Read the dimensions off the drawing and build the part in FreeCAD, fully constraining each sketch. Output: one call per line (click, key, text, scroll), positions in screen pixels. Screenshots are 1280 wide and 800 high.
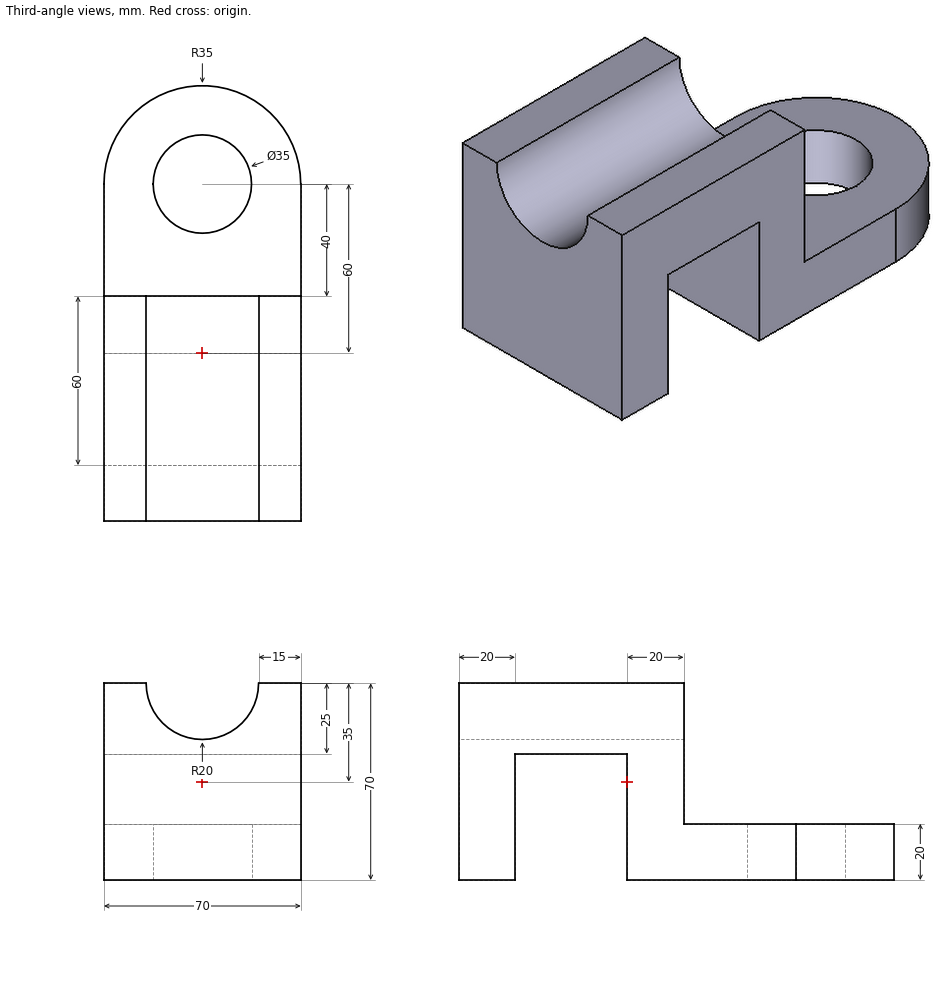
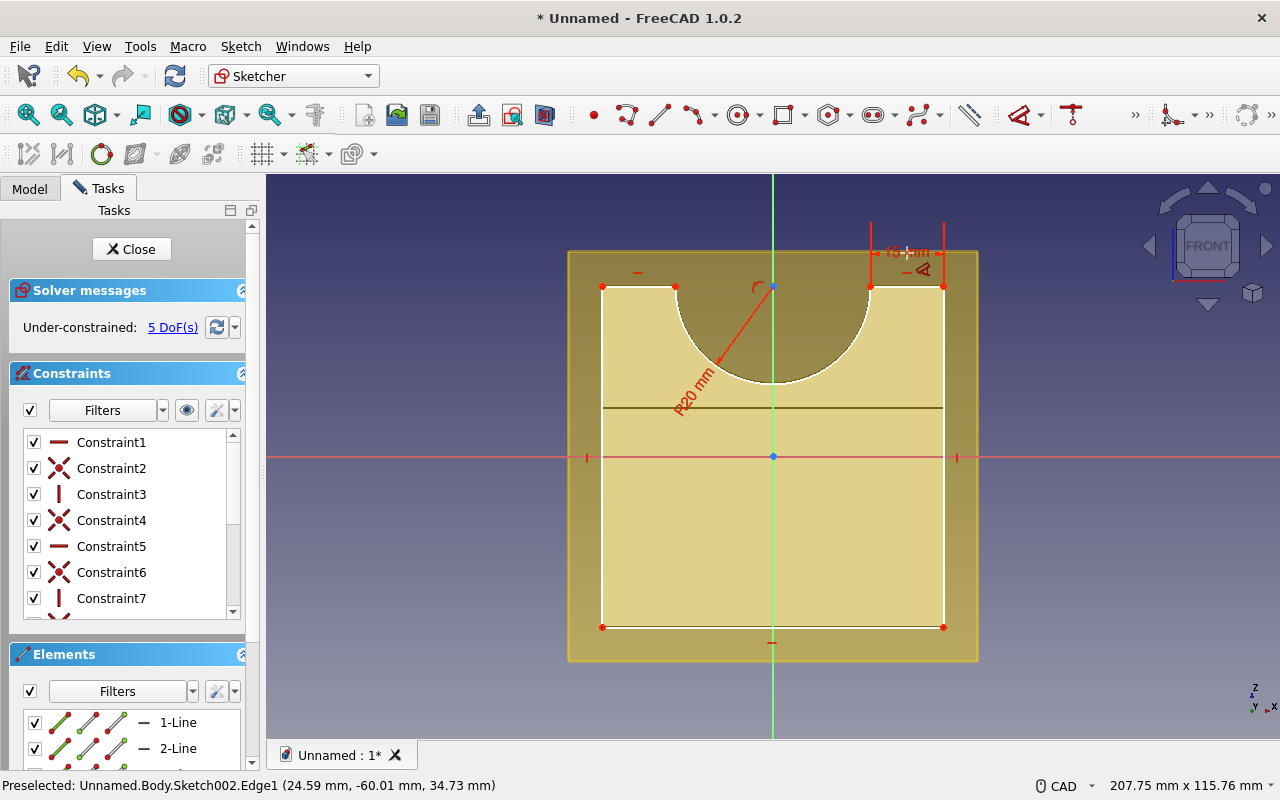
click(944, 389)
click(978, 379)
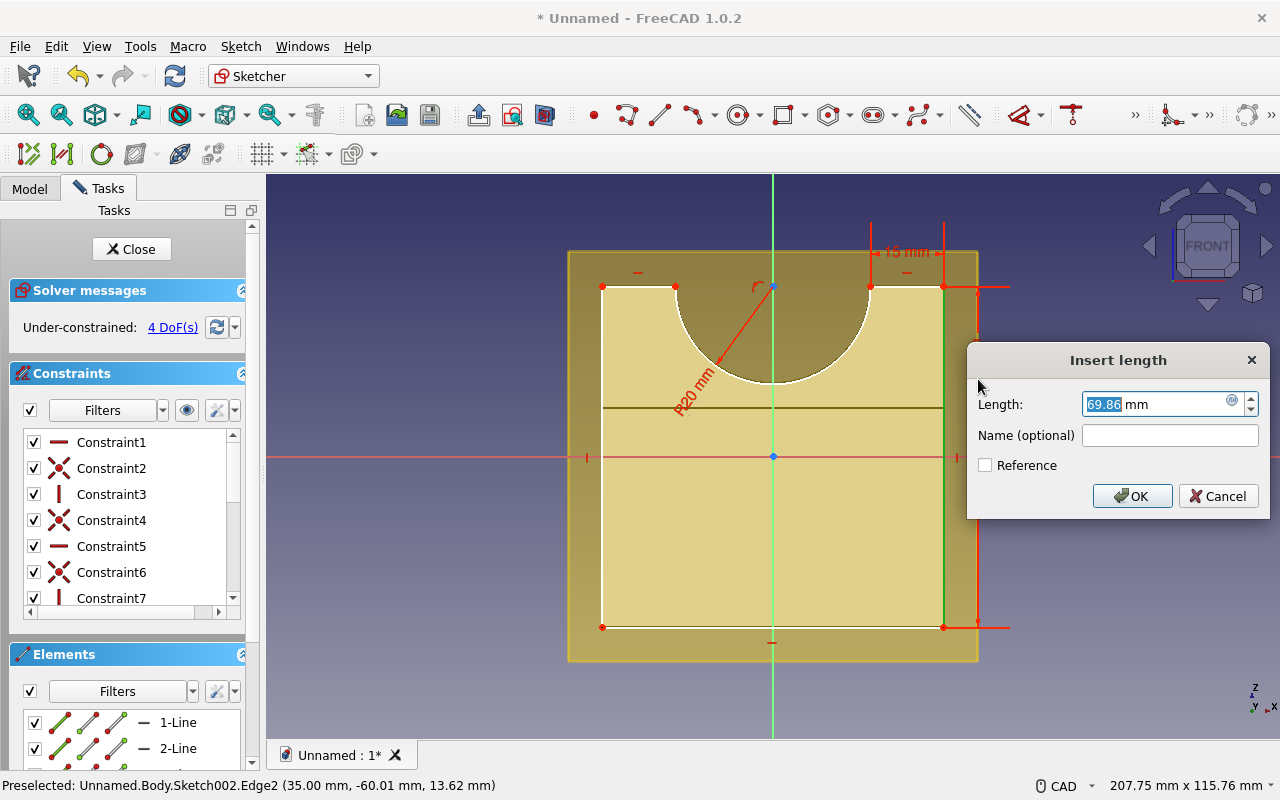
text(70)
key(Return)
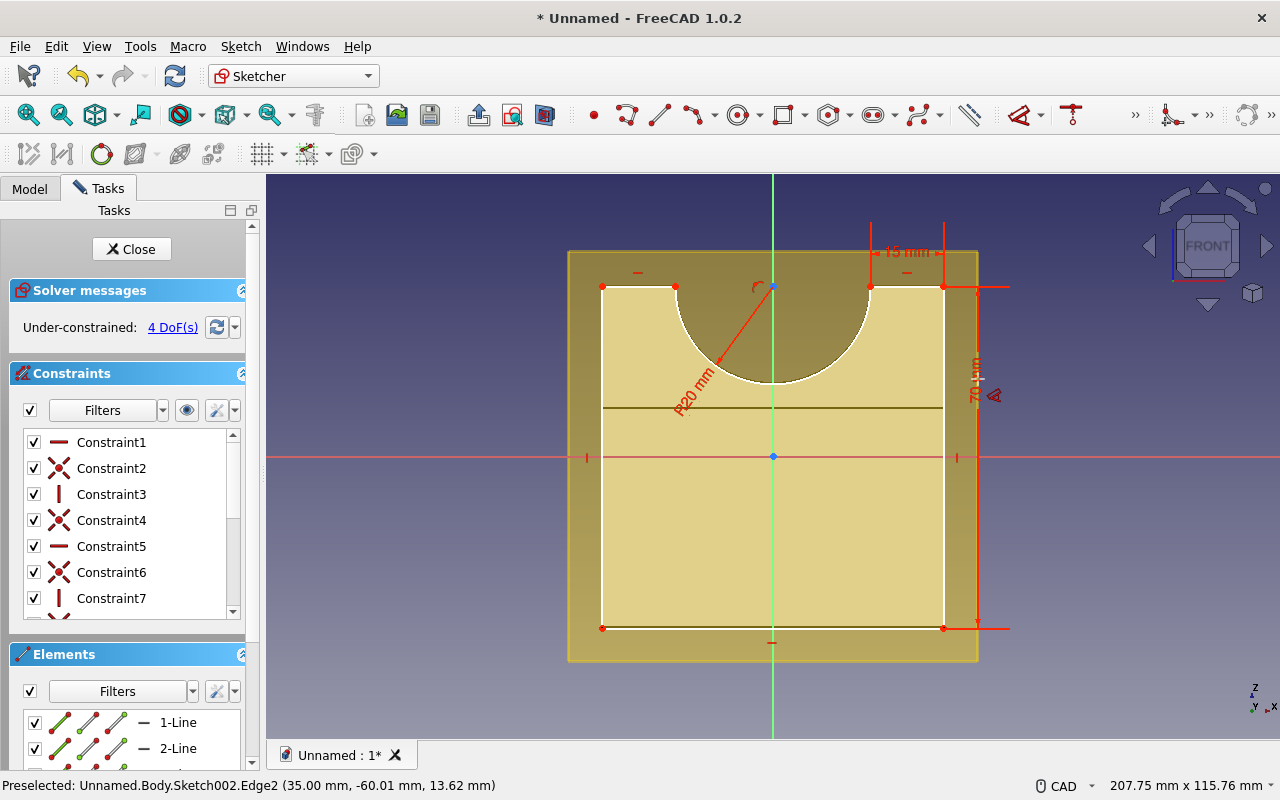
click(841, 629)
click(694, 663)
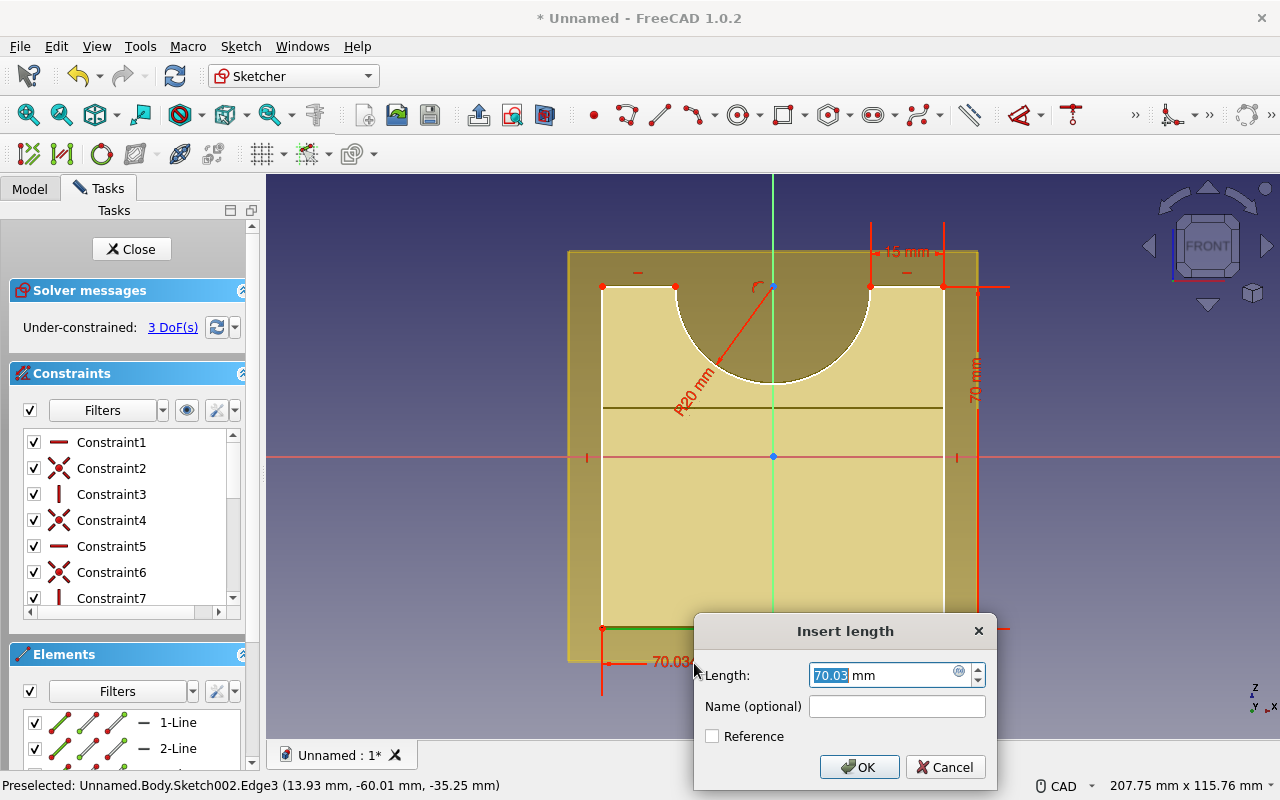
text(70)
key(Return)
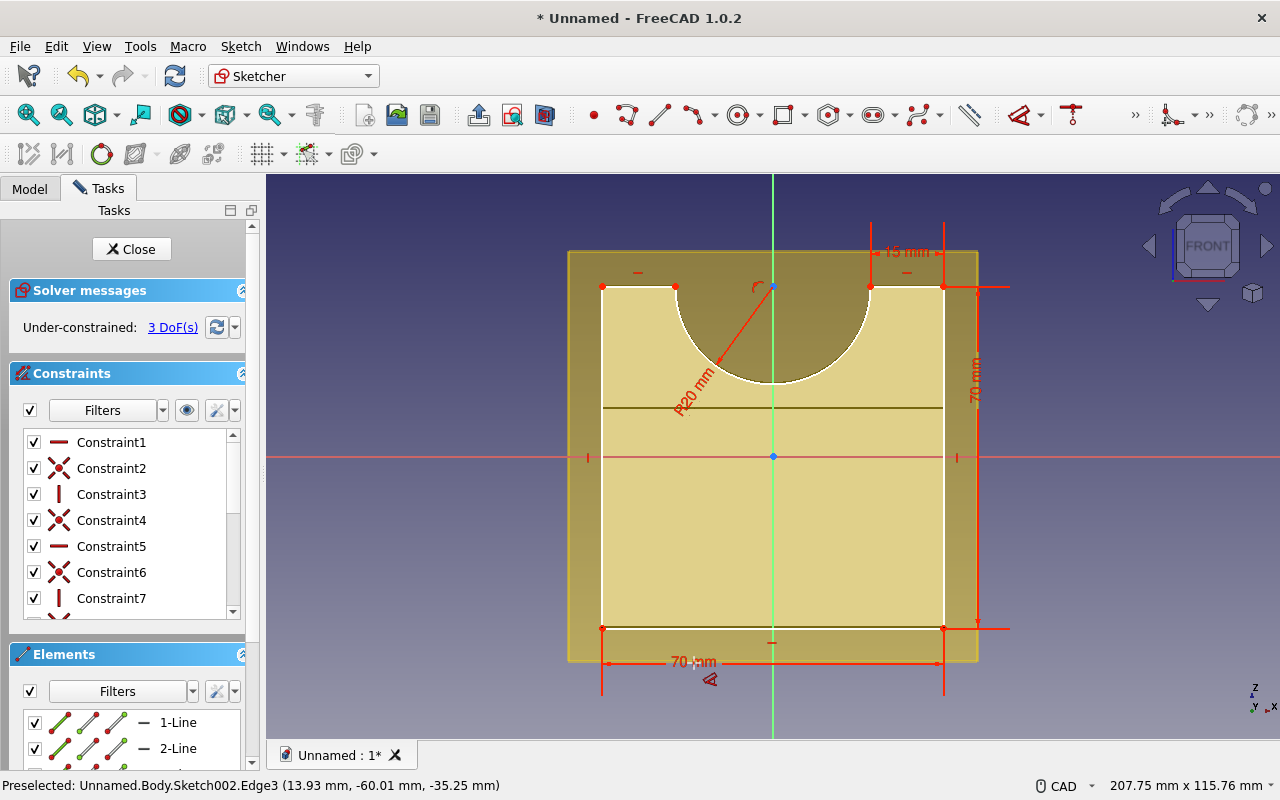
click(602, 526)
click(568, 379)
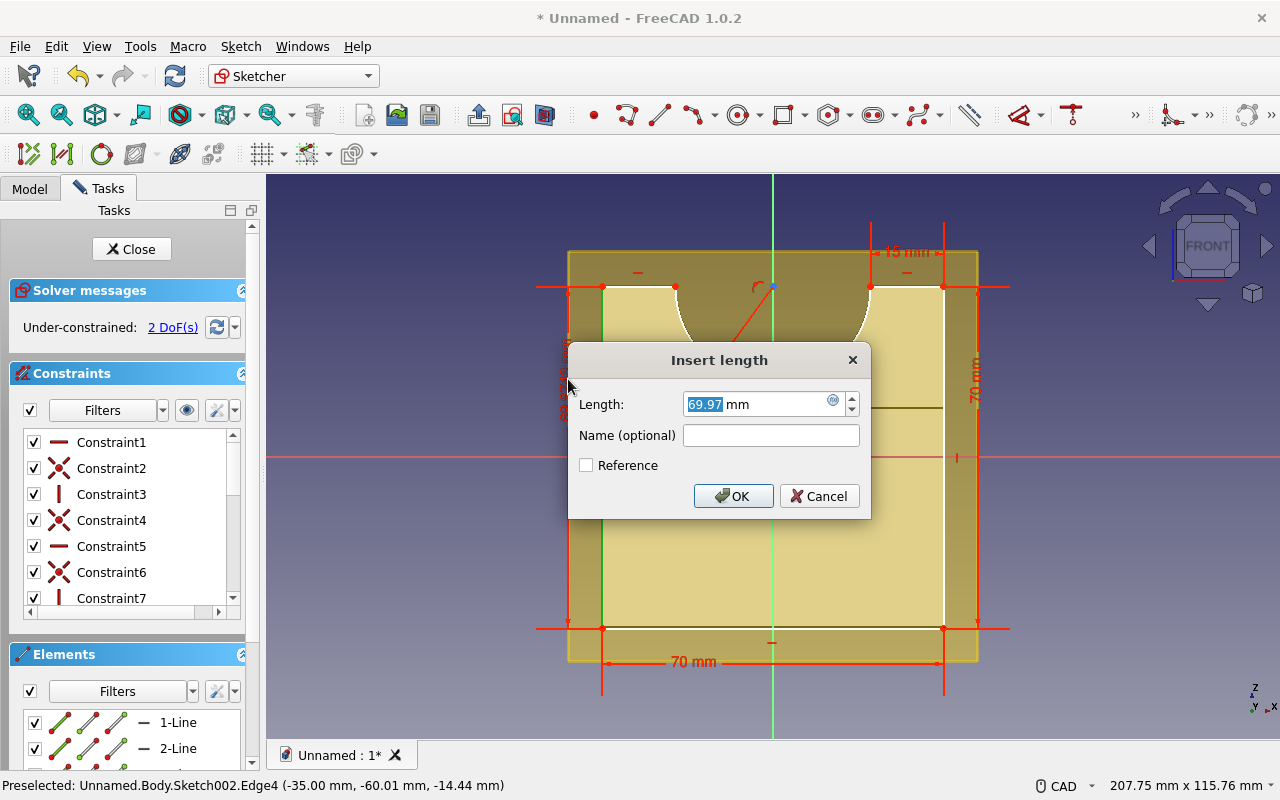
text(70)
key(Return)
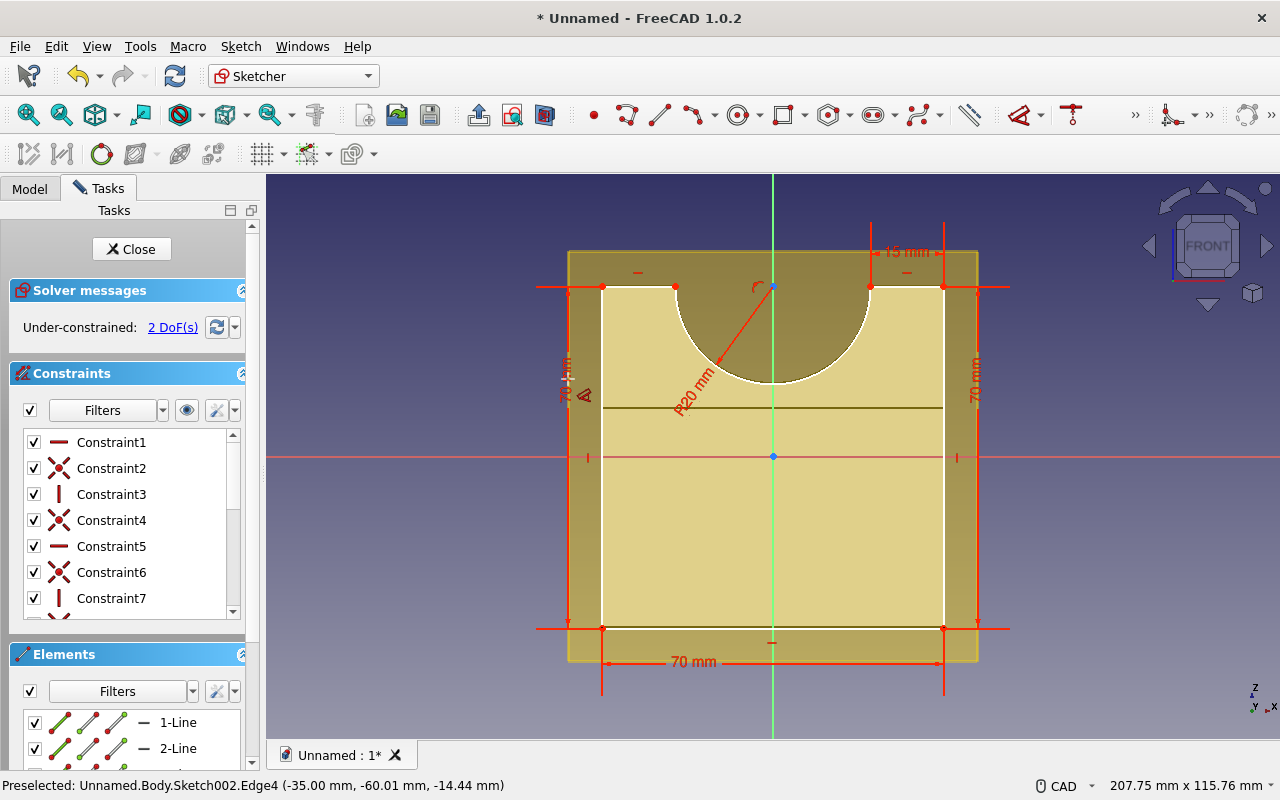
click(871, 287)
click(905, 372)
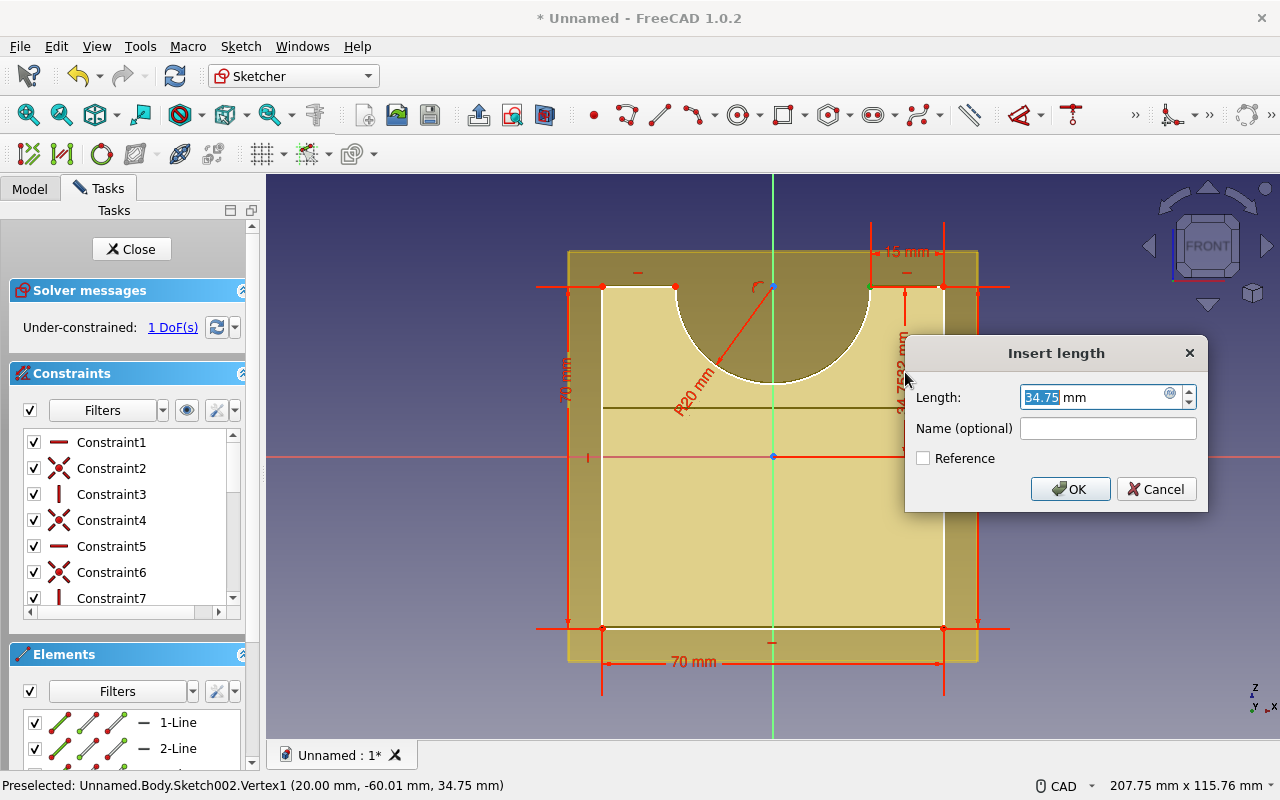
text(35)
key(Return)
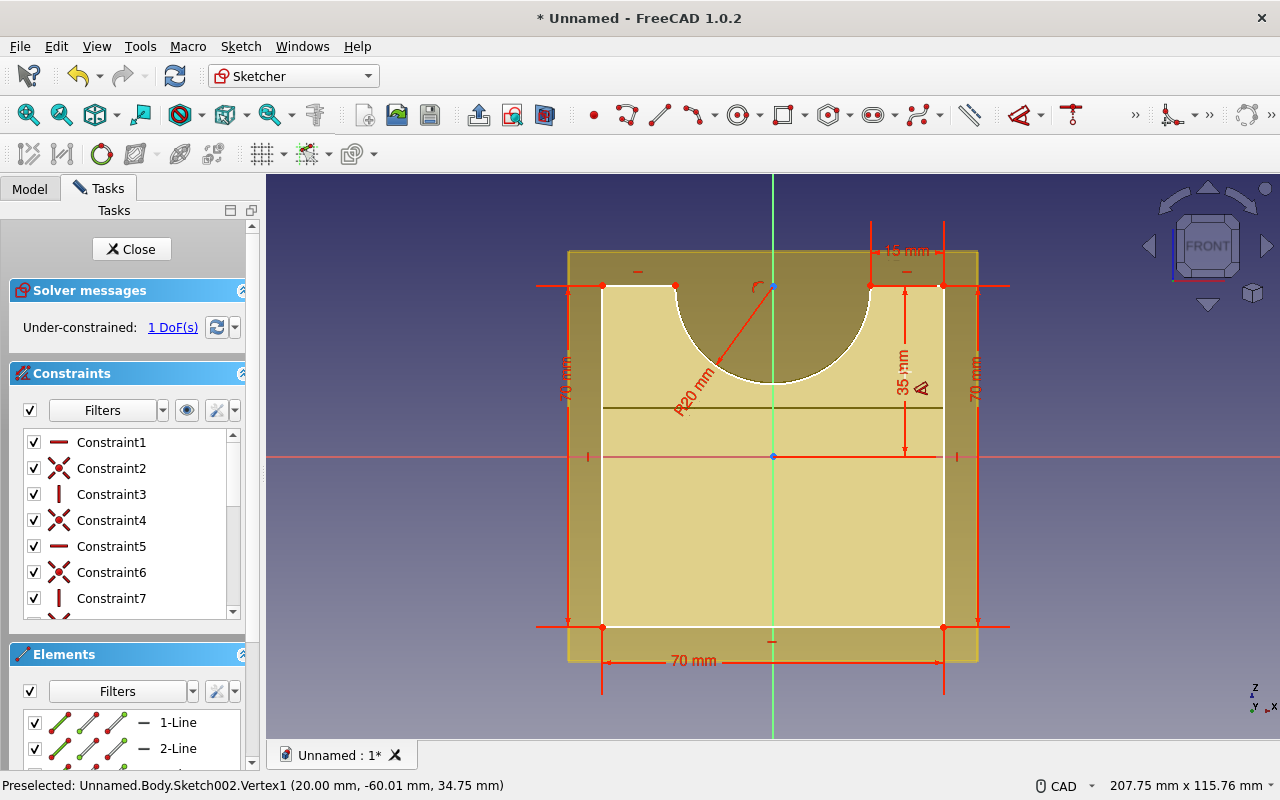
click(773, 287)
click(807, 333)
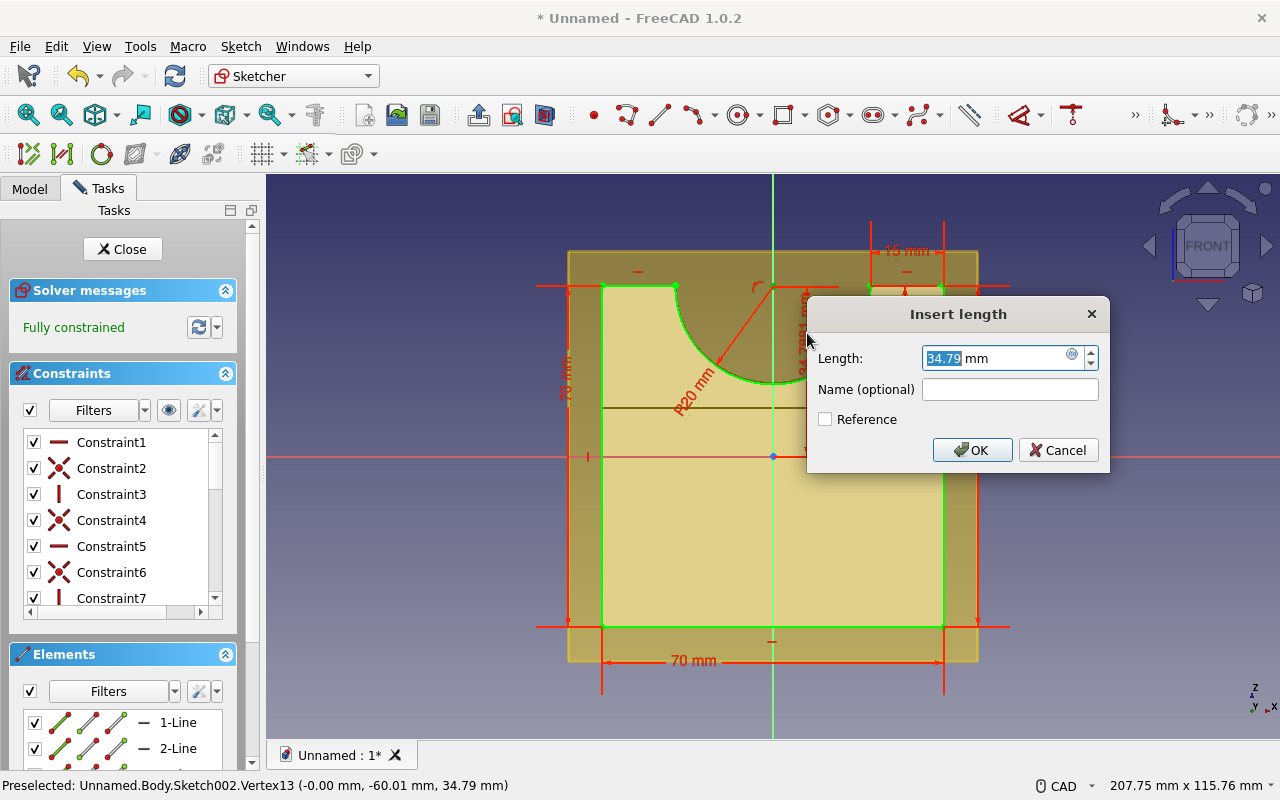
text(35)
key(Return)
key(Escape)